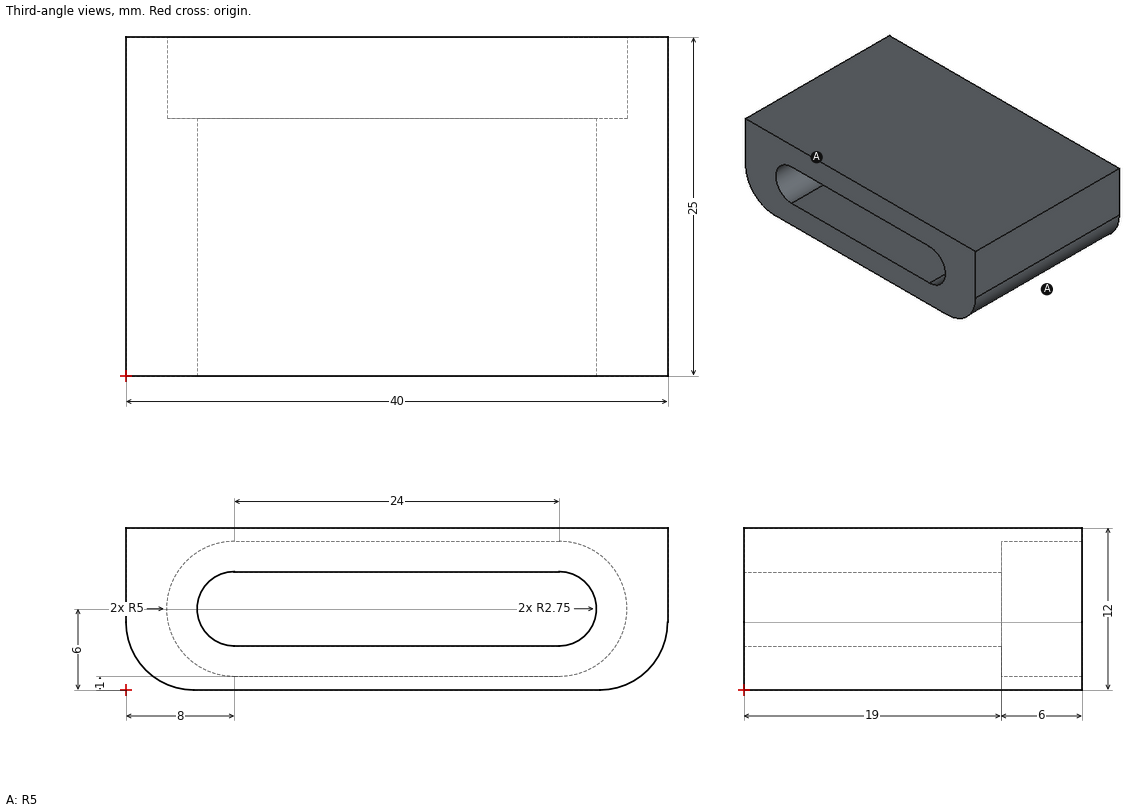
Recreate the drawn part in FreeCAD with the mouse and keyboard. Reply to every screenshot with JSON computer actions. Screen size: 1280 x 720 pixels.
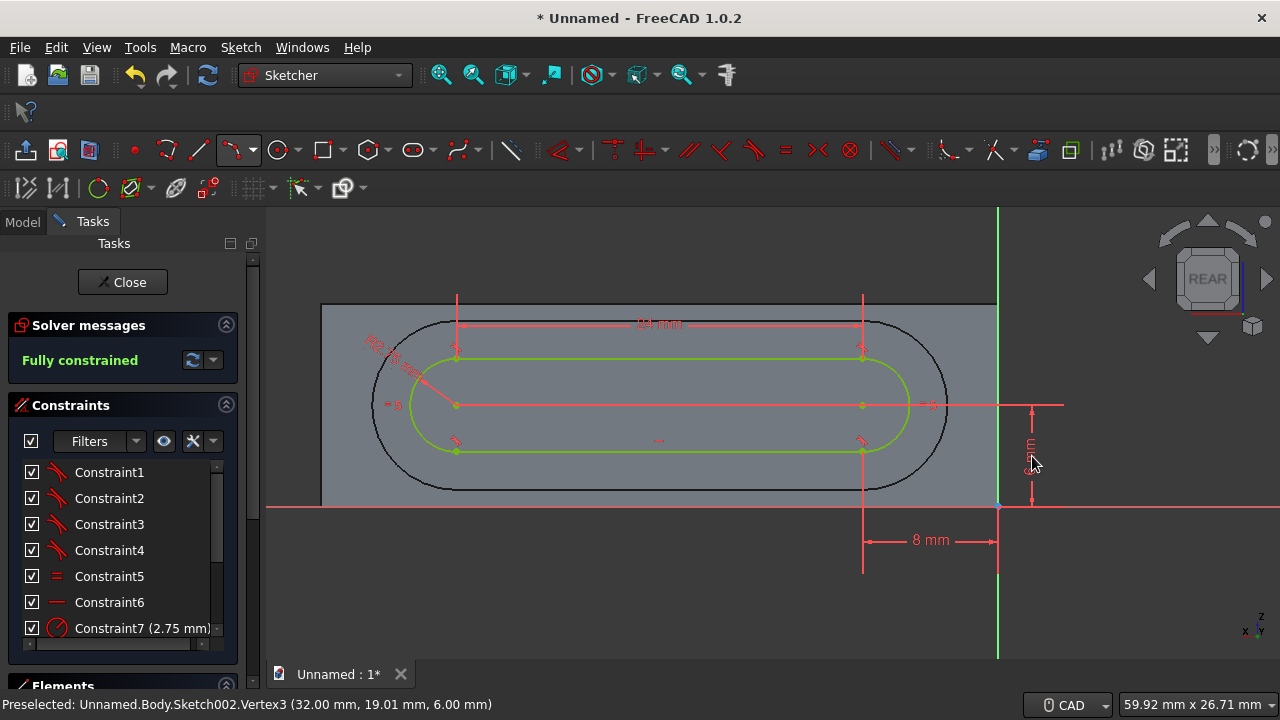
{"action": "left_click", "coordinate": [123, 282]}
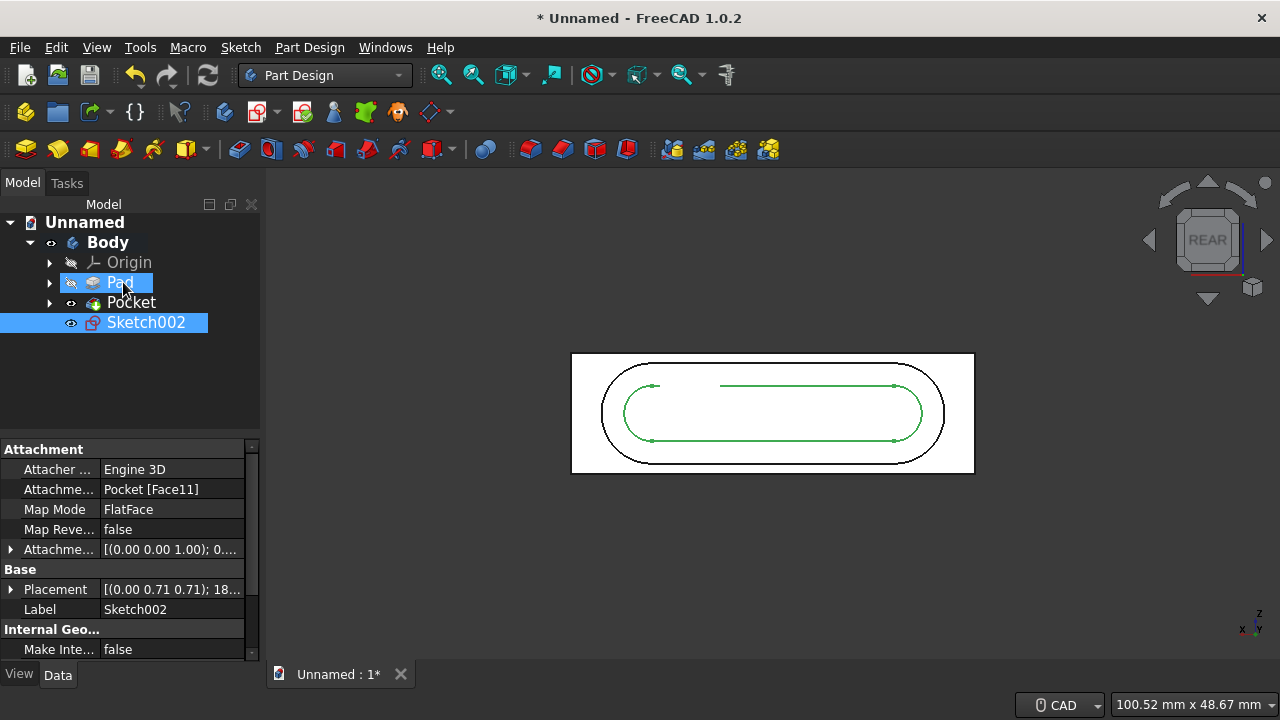
{"action": "left_click", "coordinate": [240, 150]}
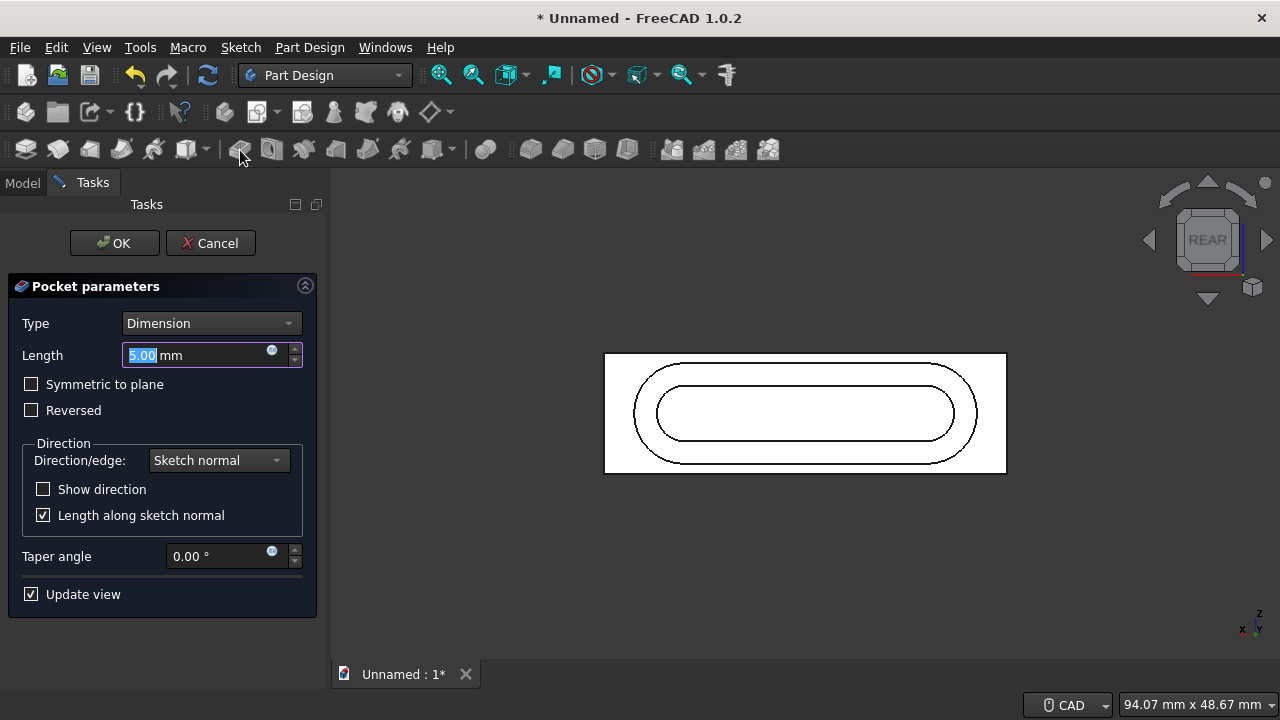
{"action": "type", "text": "19"}
{"action": "key", "text": "Tab"}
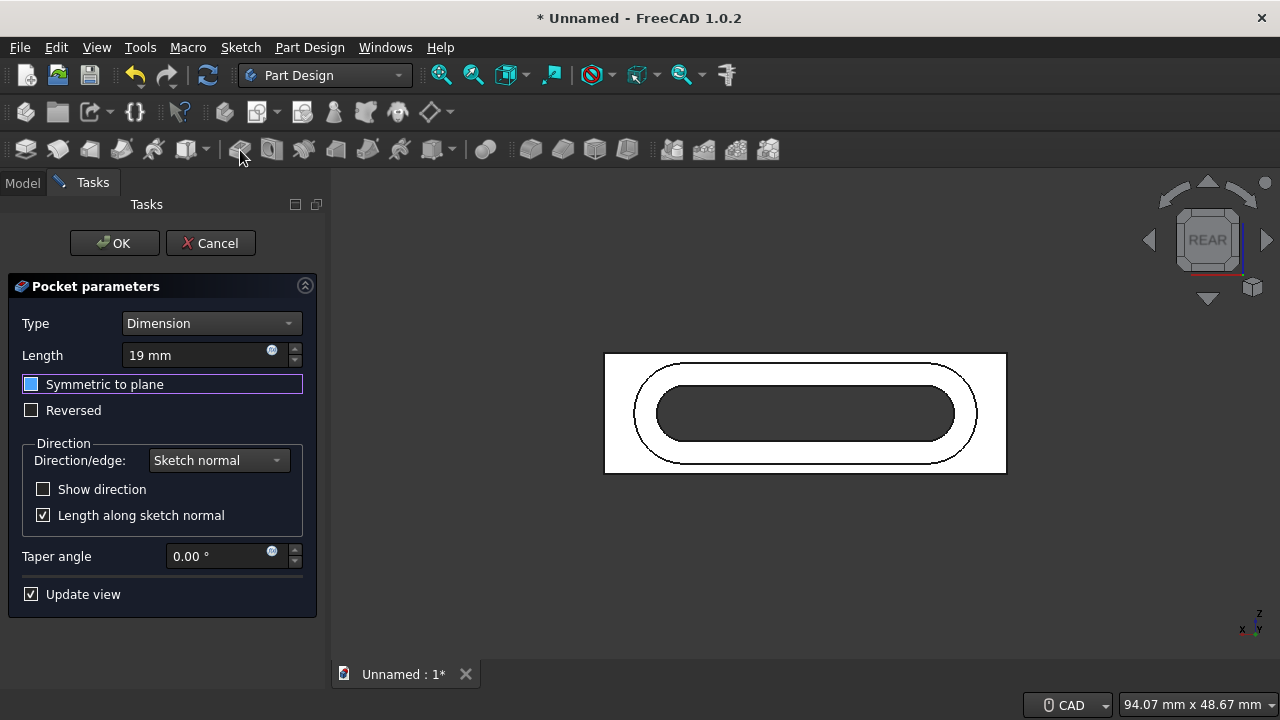
{"action": "left_click", "coordinate": [115, 243]}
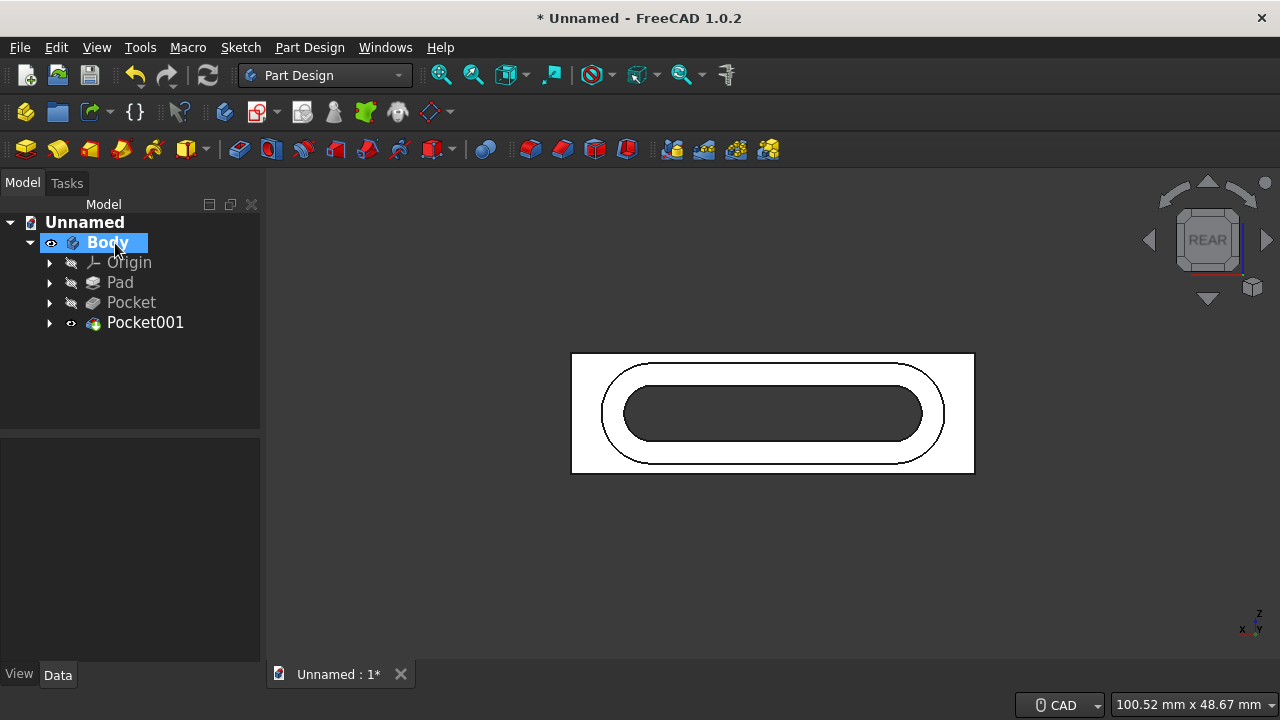
{"action": "key", "text": "v f"}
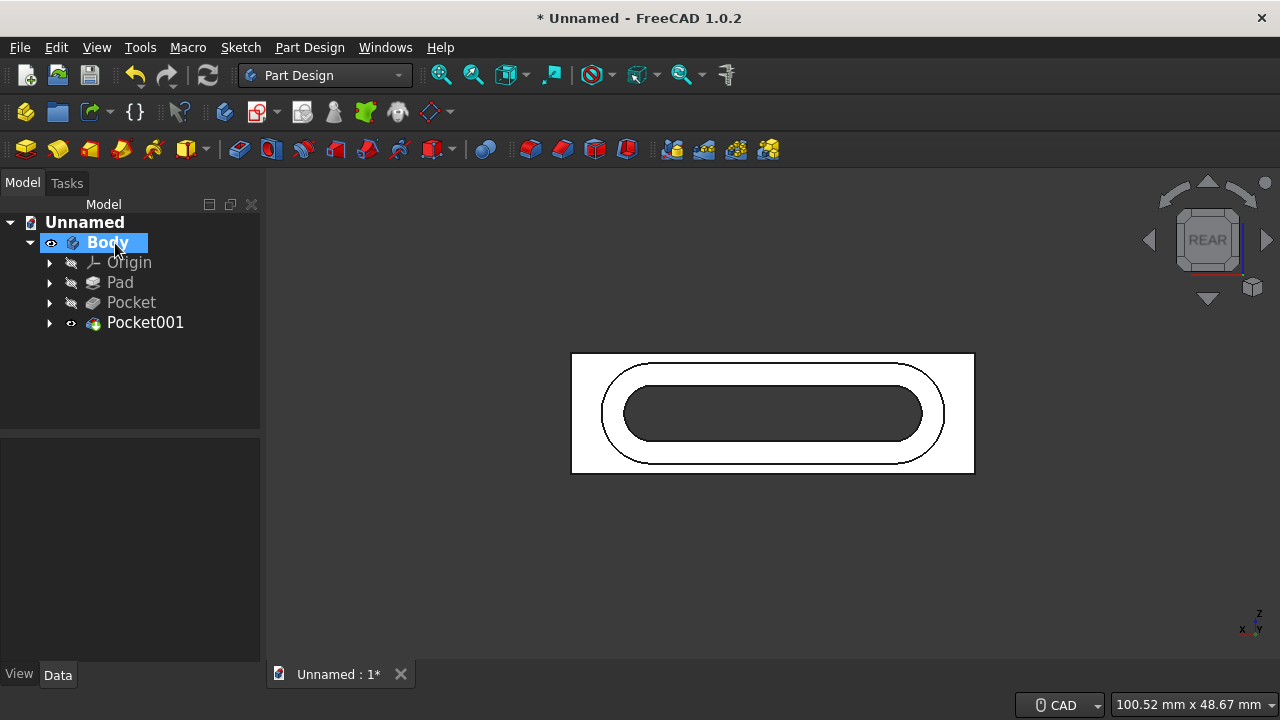
{"action": "key", "text": "0"}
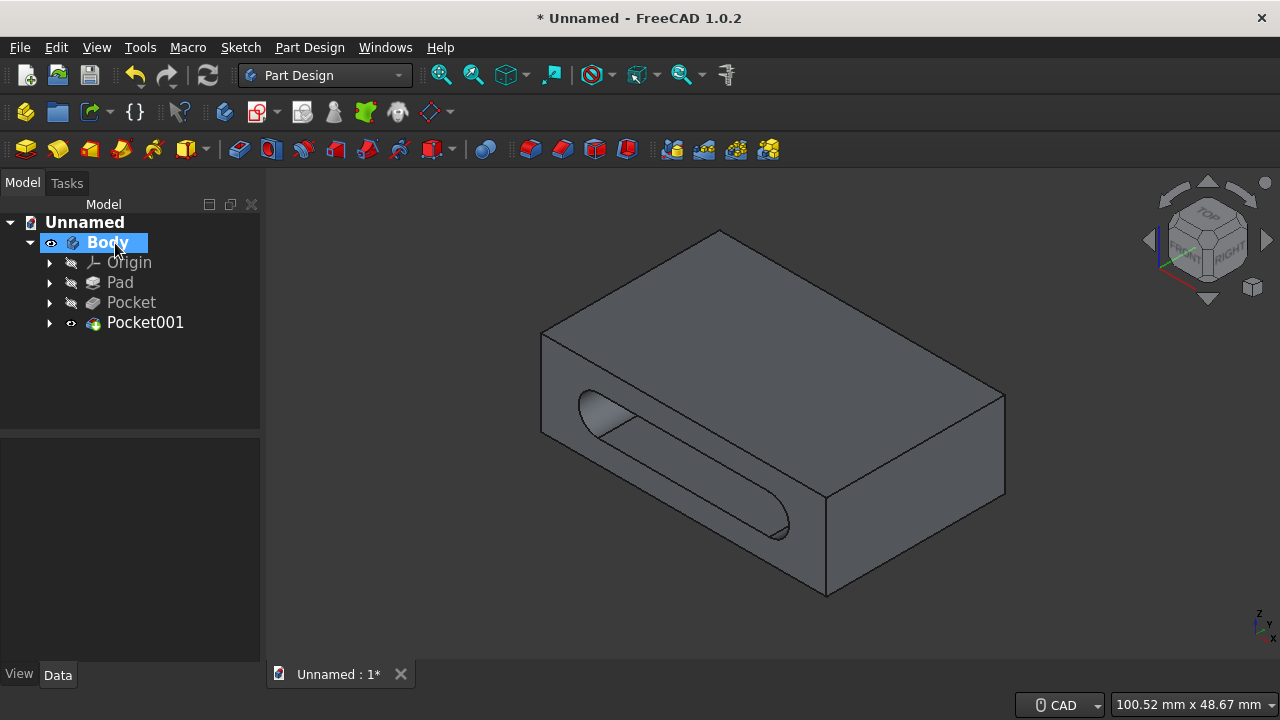
{"action": "key", "text": "2"}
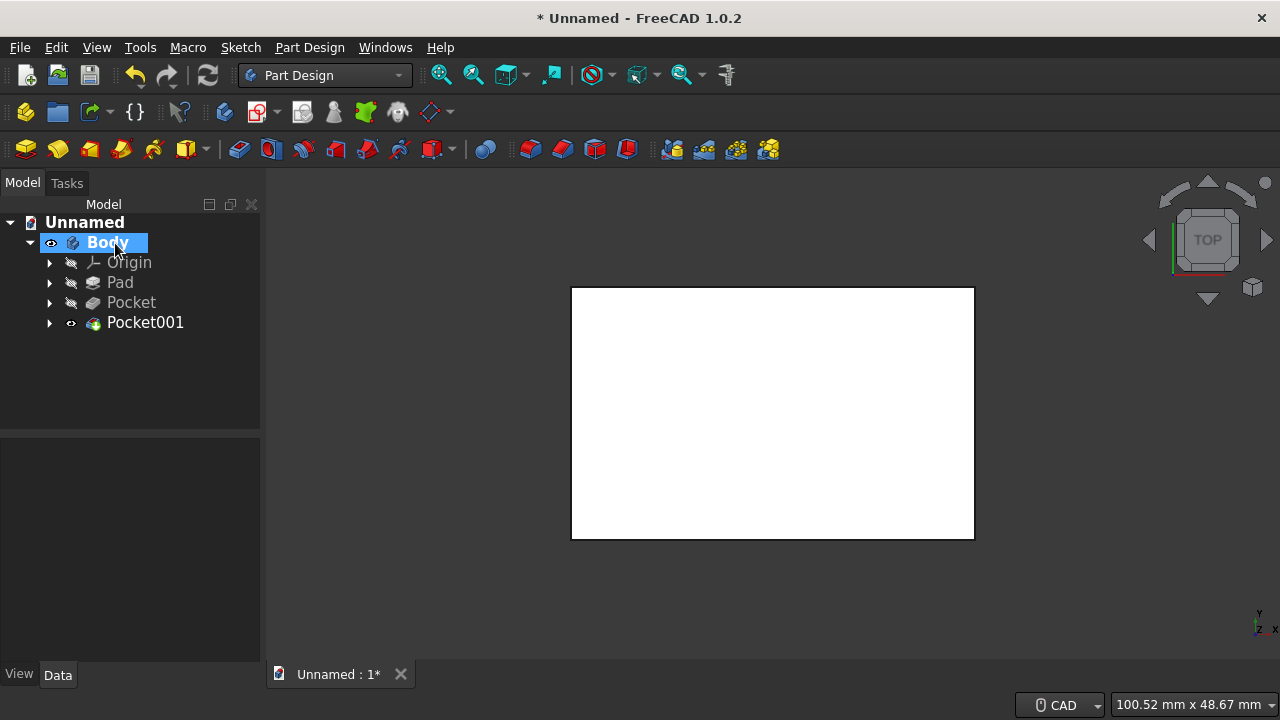
{"action": "key", "text": "1"}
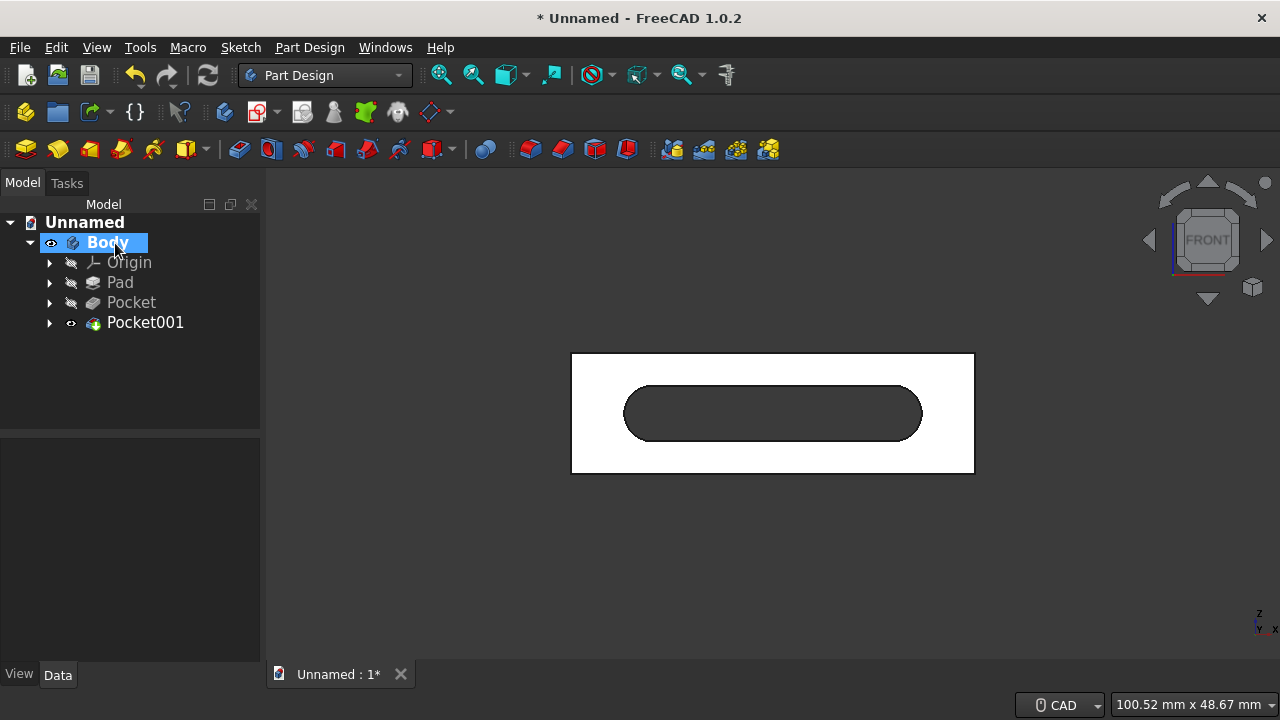
{"action": "key", "text": "v f"}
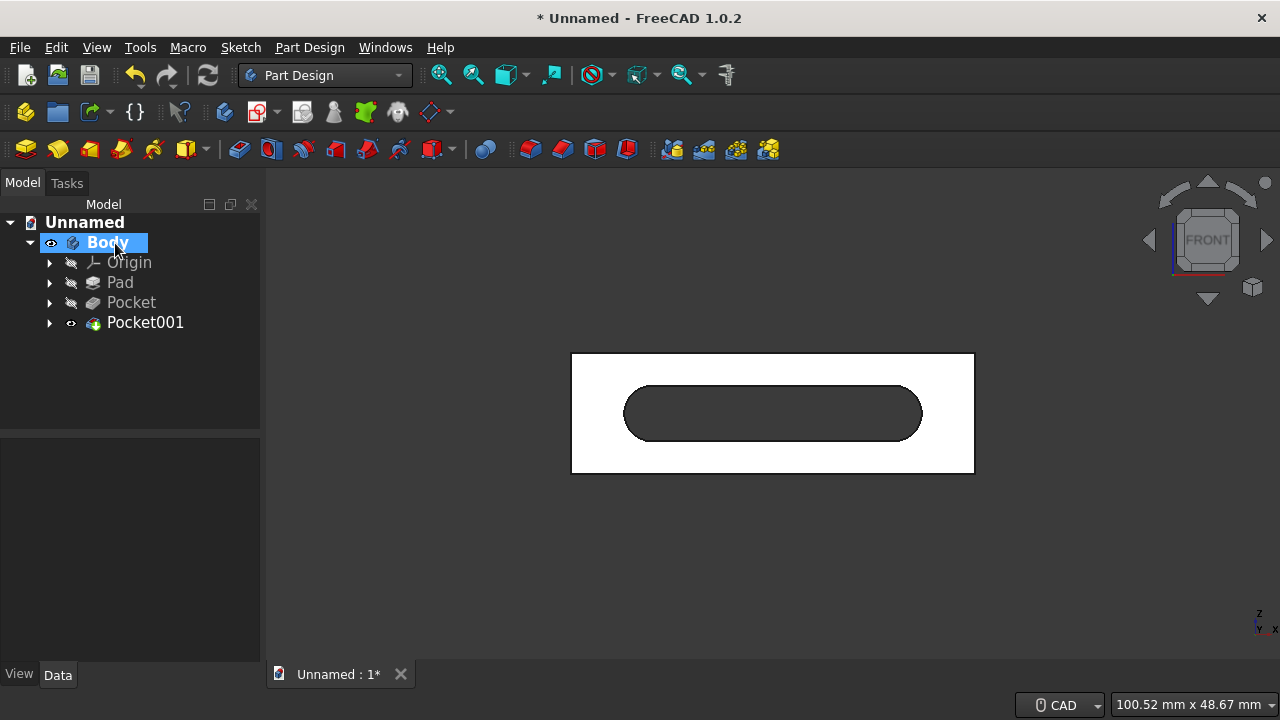
{"action": "key", "text": "3"}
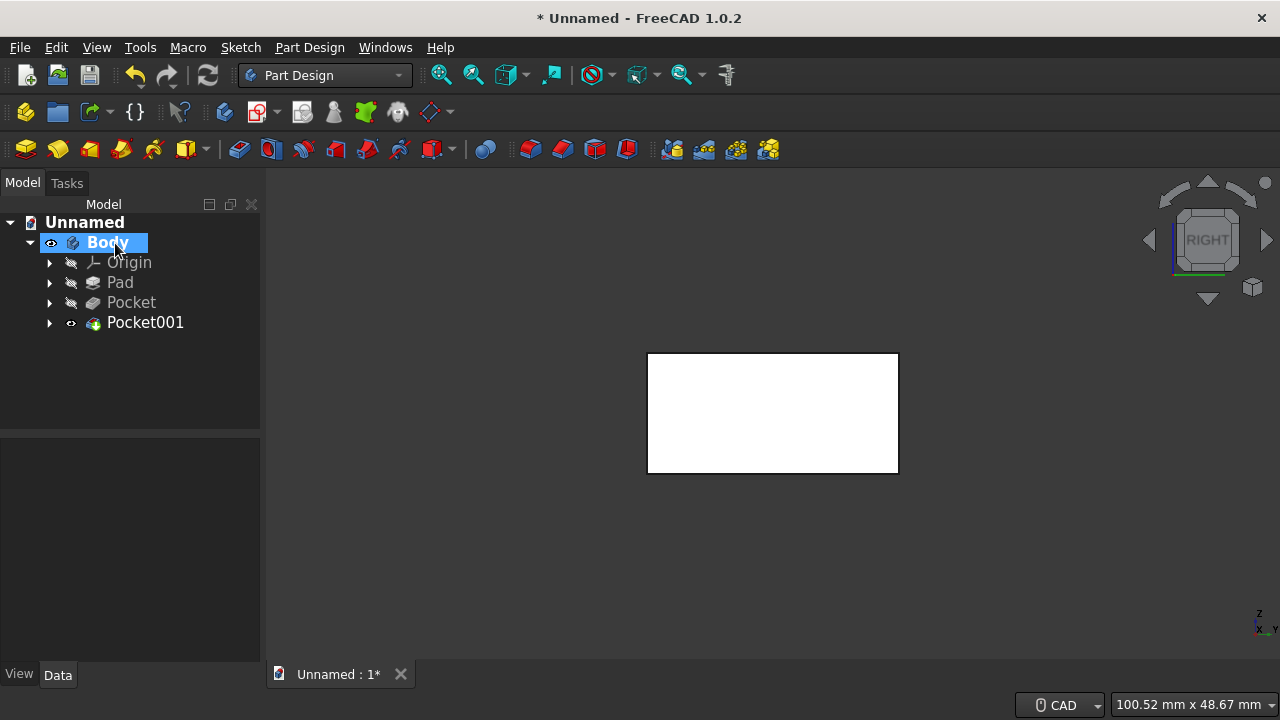
{"action": "key", "text": "v f"}